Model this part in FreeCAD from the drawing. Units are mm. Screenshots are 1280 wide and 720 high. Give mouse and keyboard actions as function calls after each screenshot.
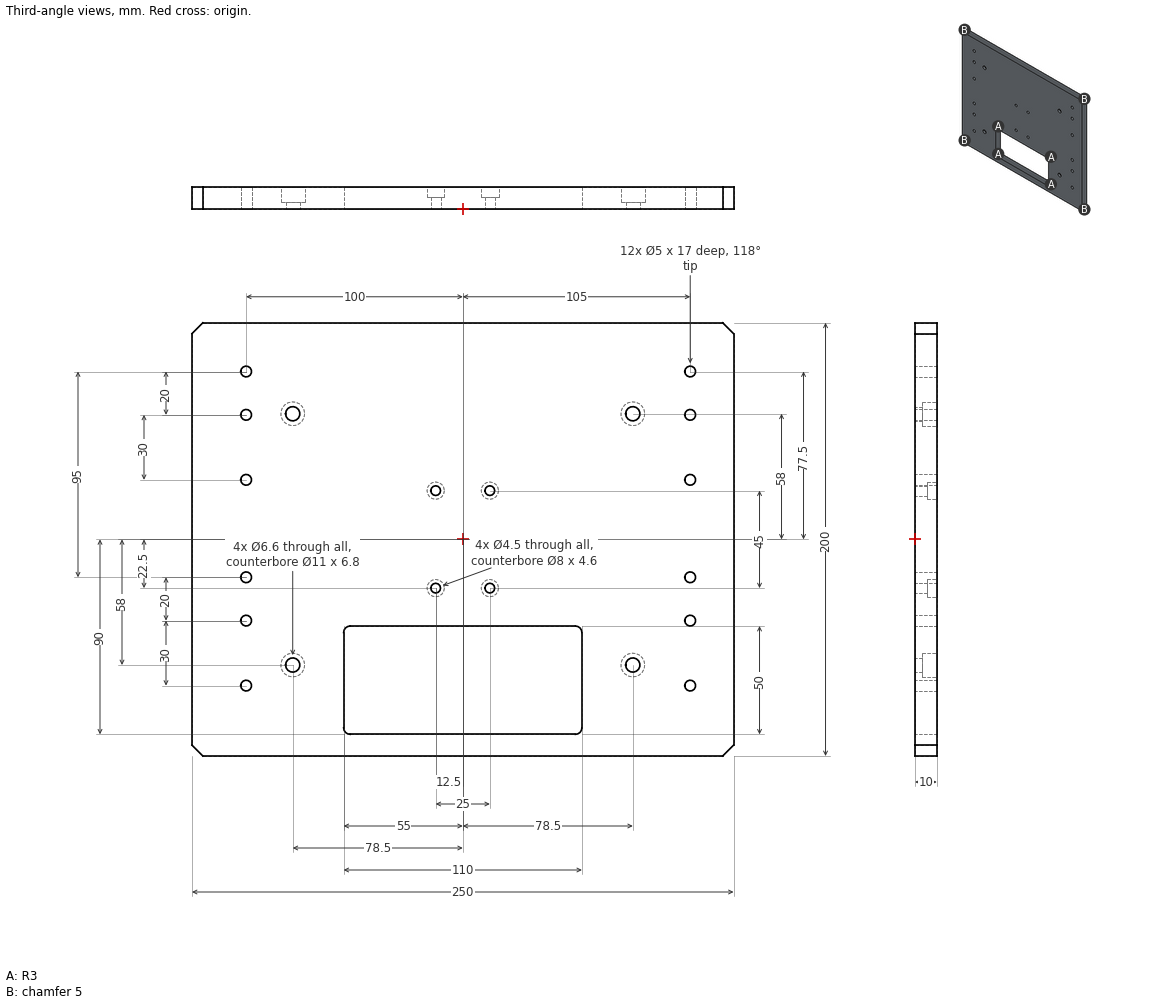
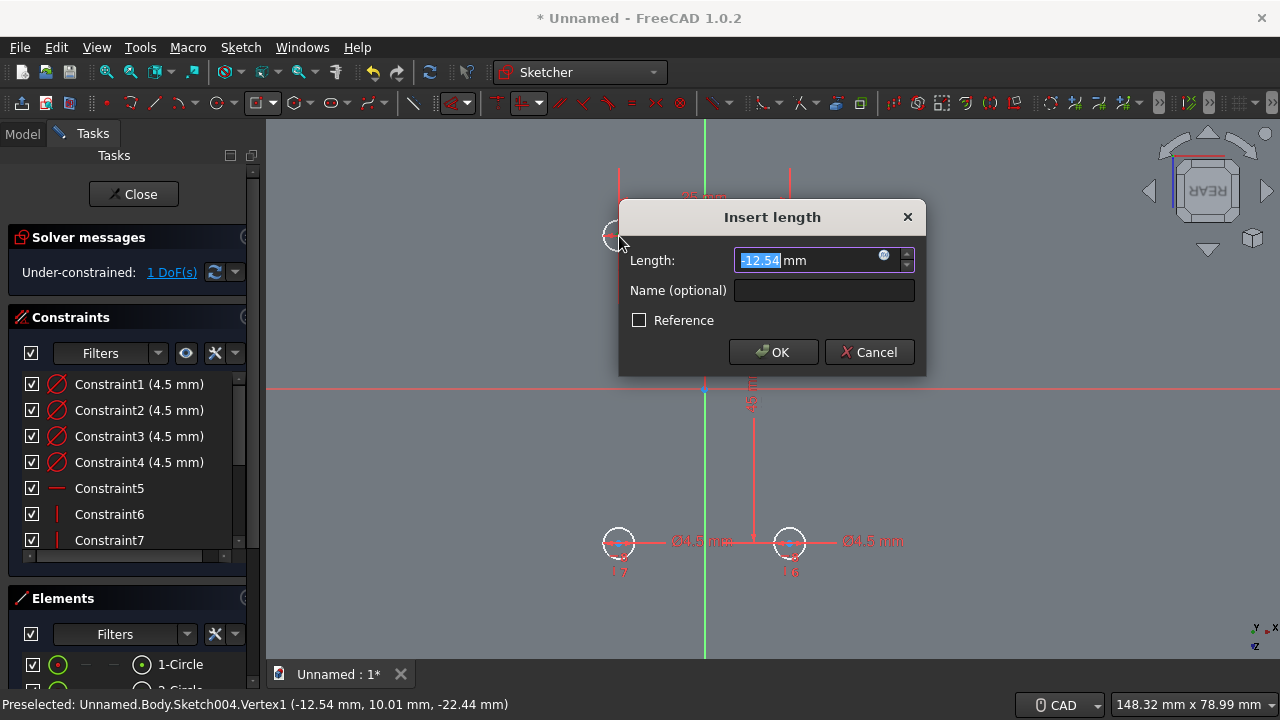
text(-12.5)
key(Return)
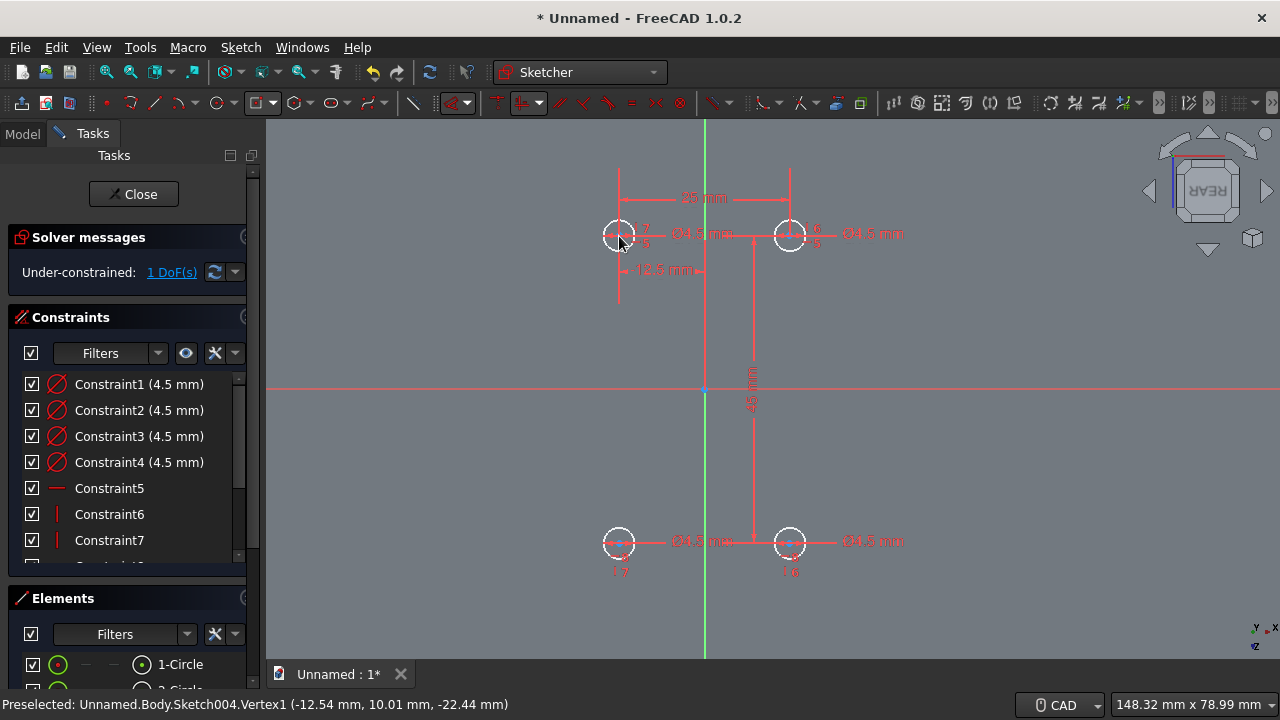
click(619, 236)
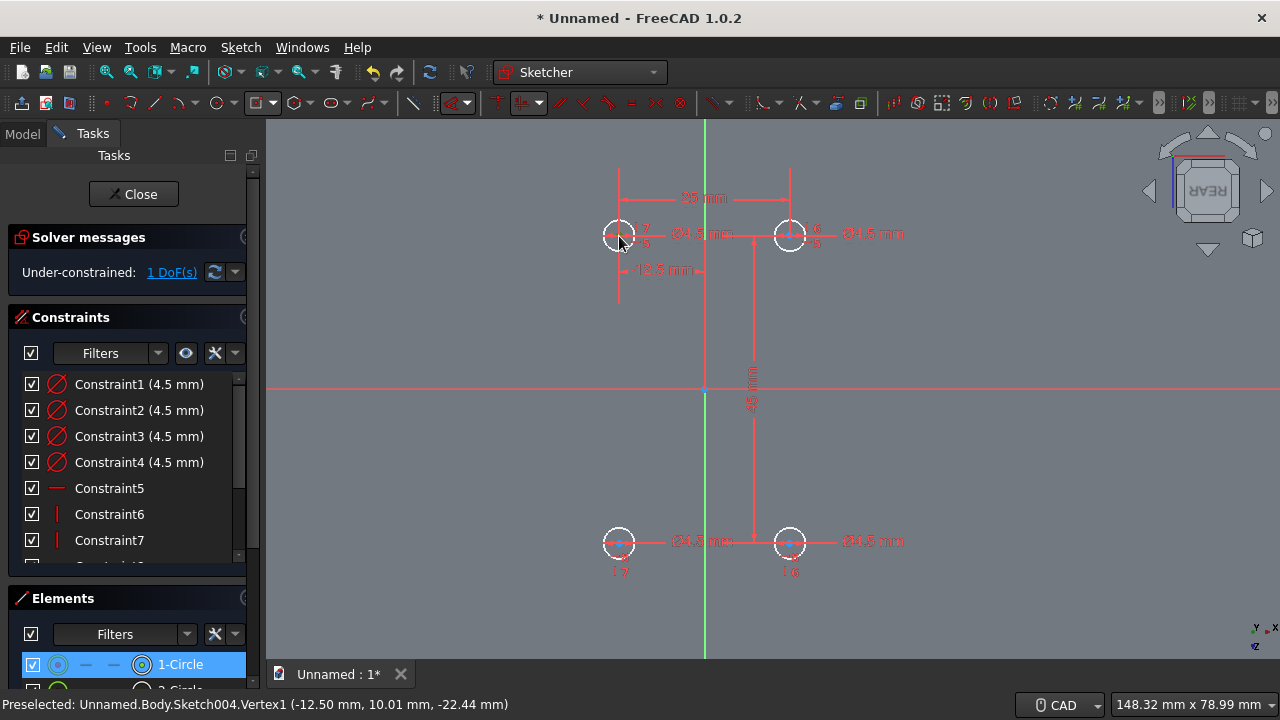
key(i)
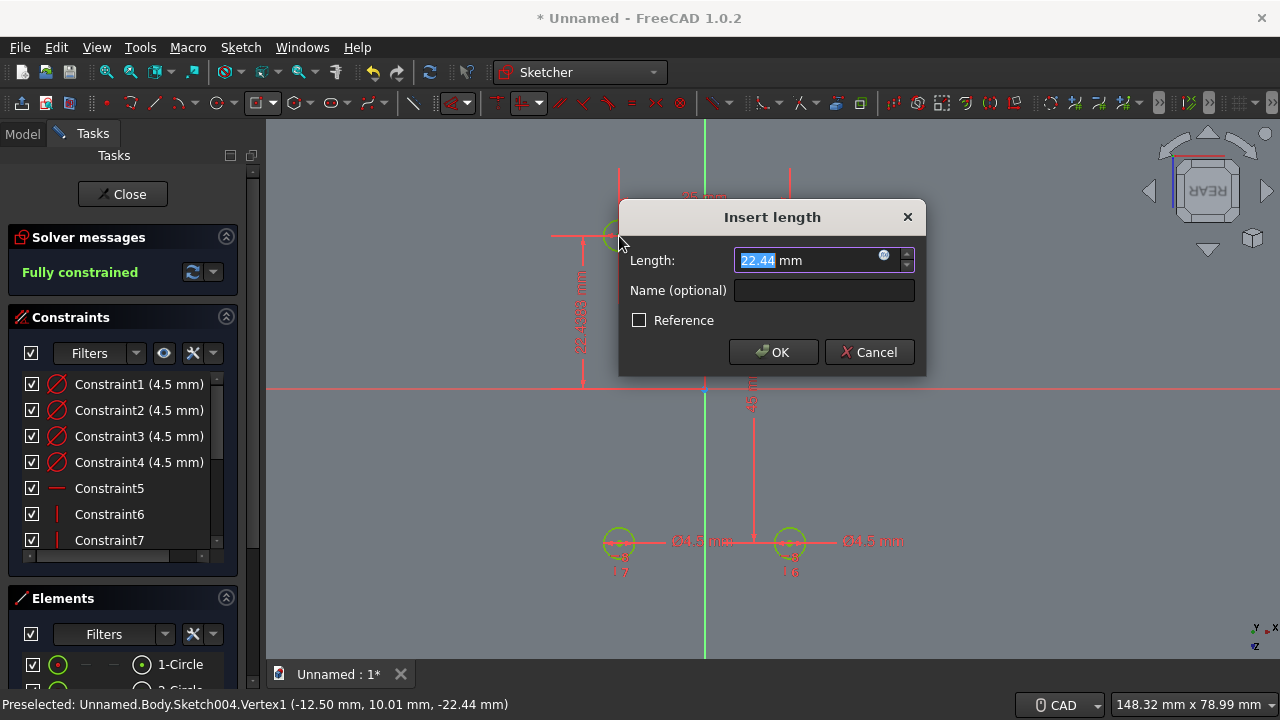
text(22.5)
key(Return)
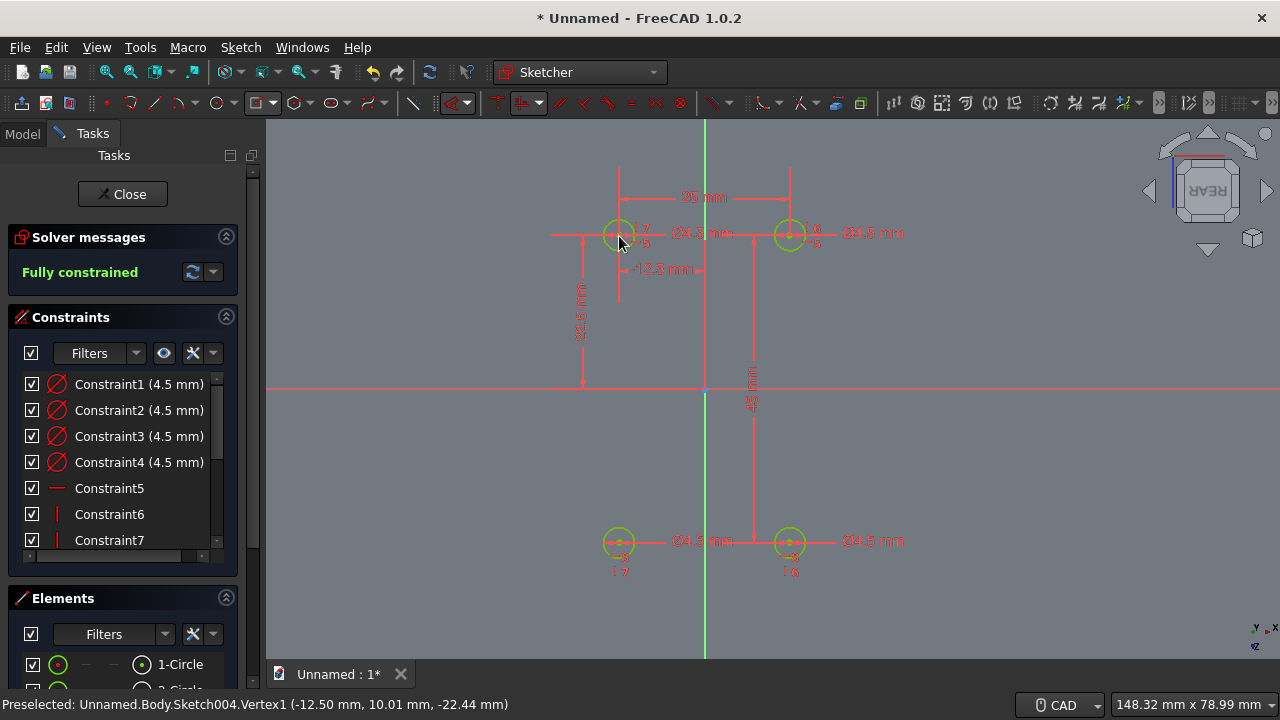
click(123, 194)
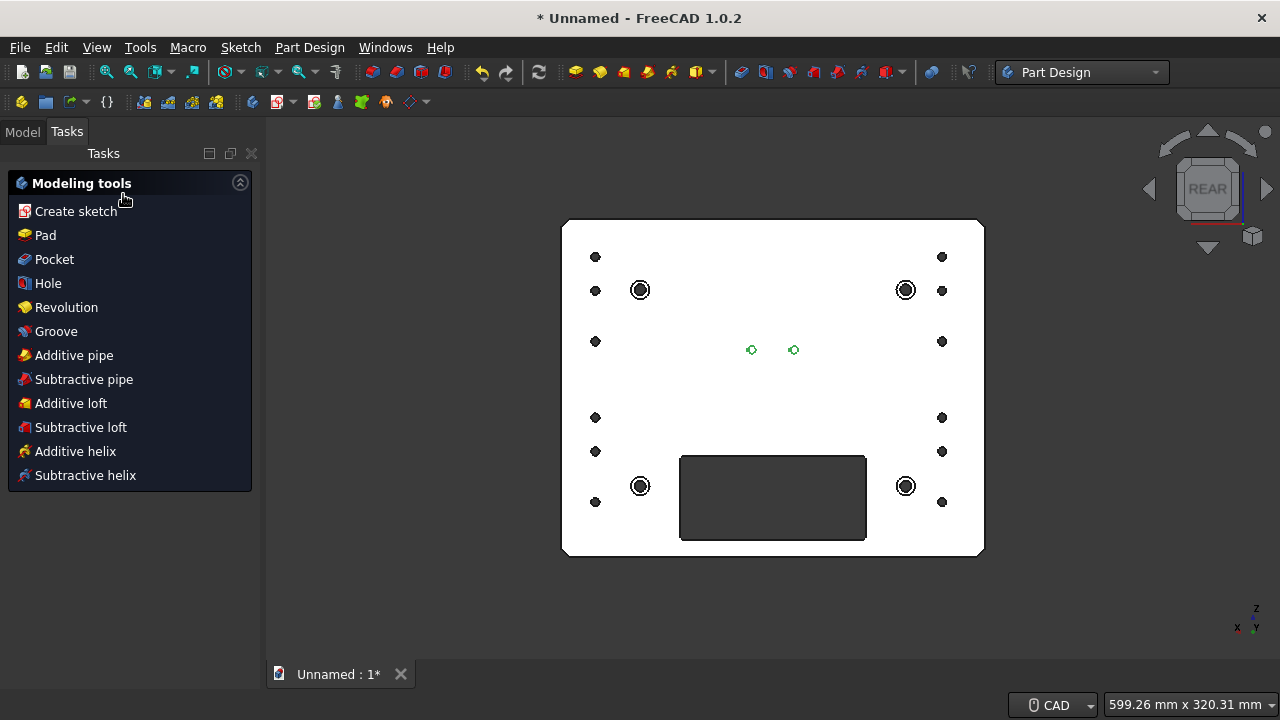
click(766, 72)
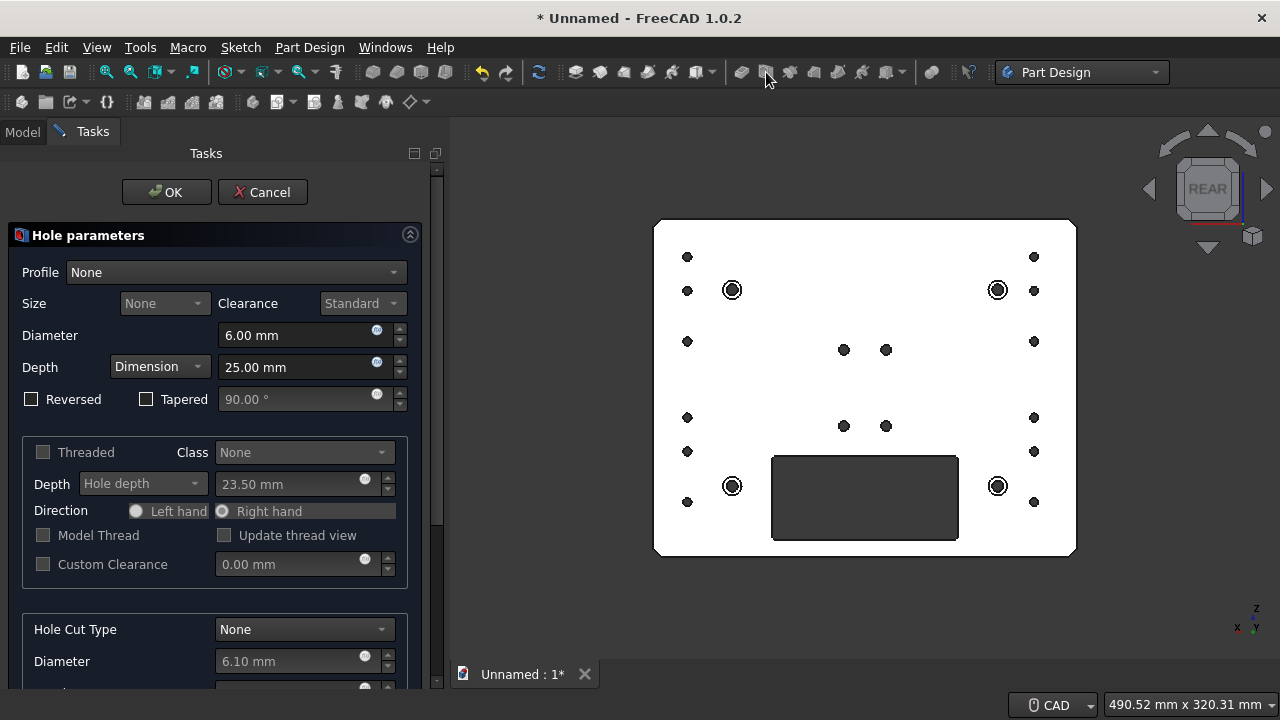
triple_click(305, 335)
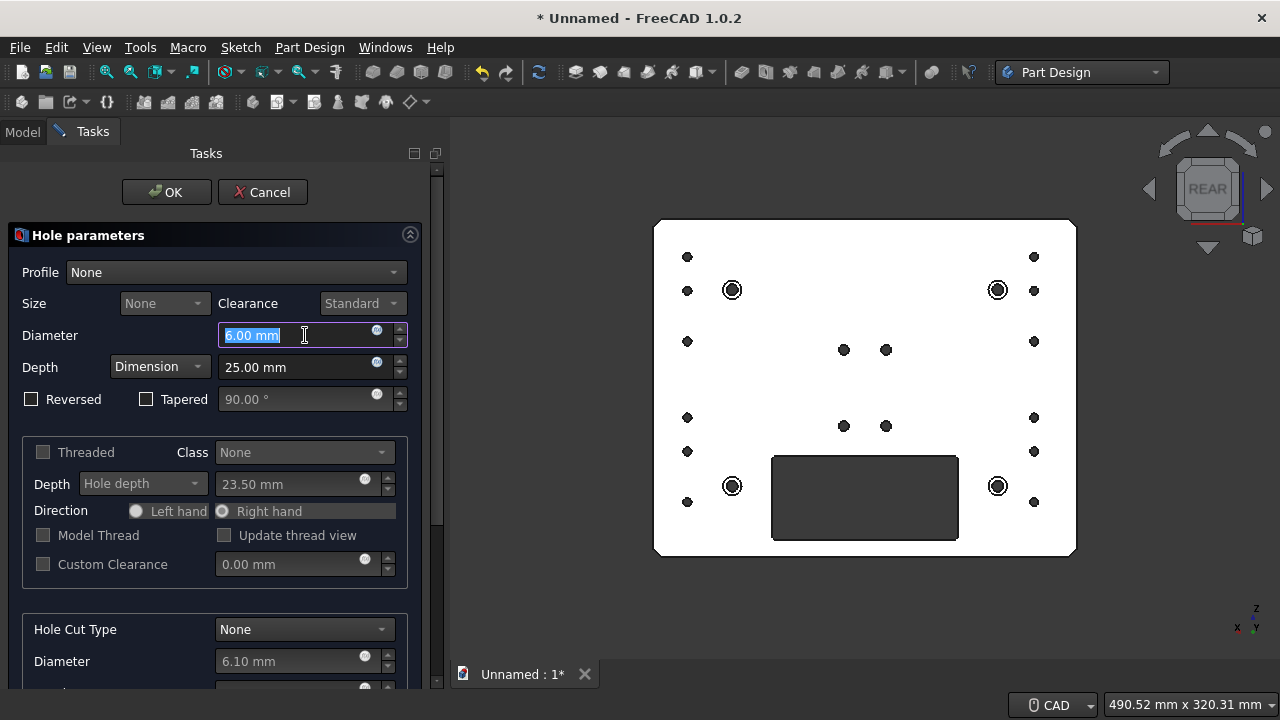
text(4.5)
key(Tab)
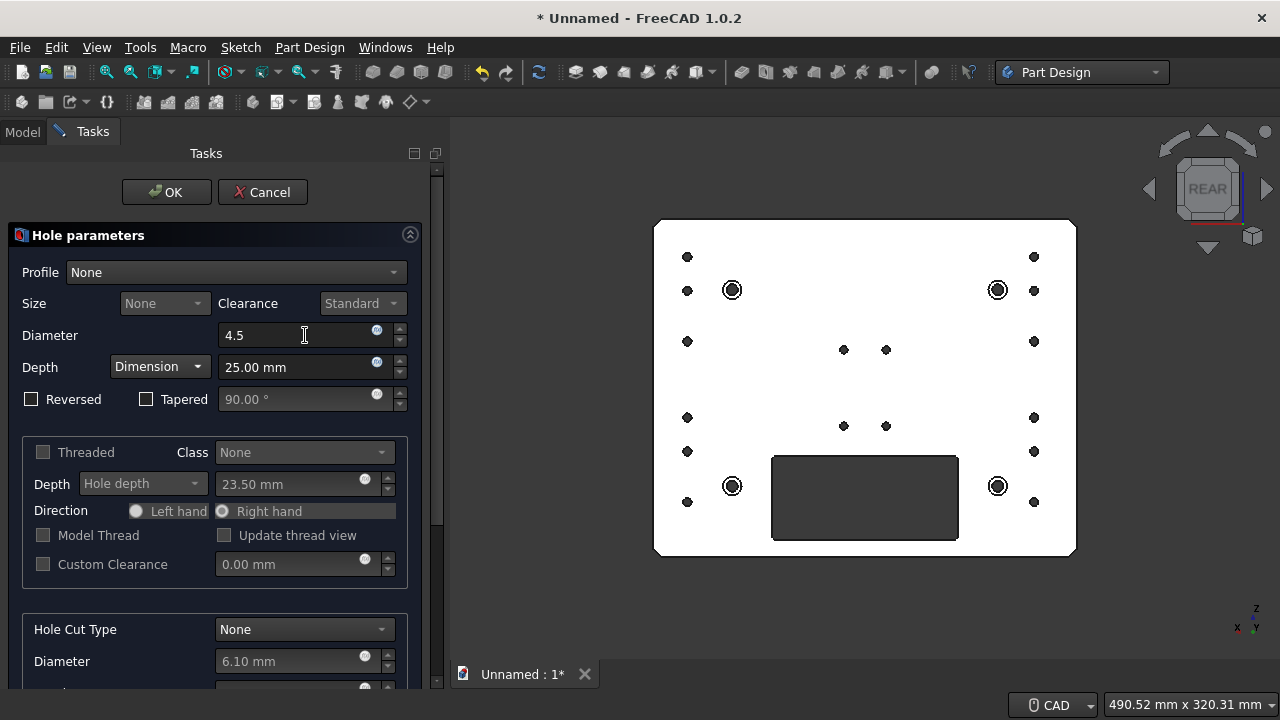
click(161, 366)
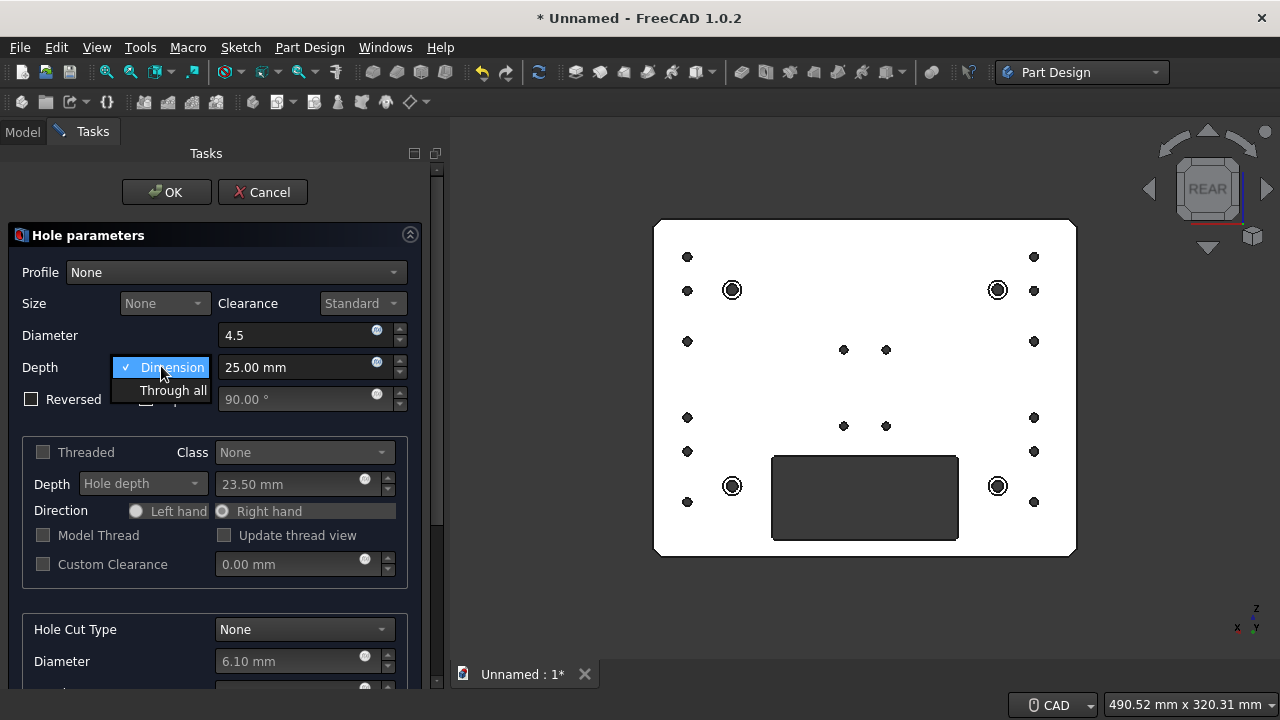
click(160, 390)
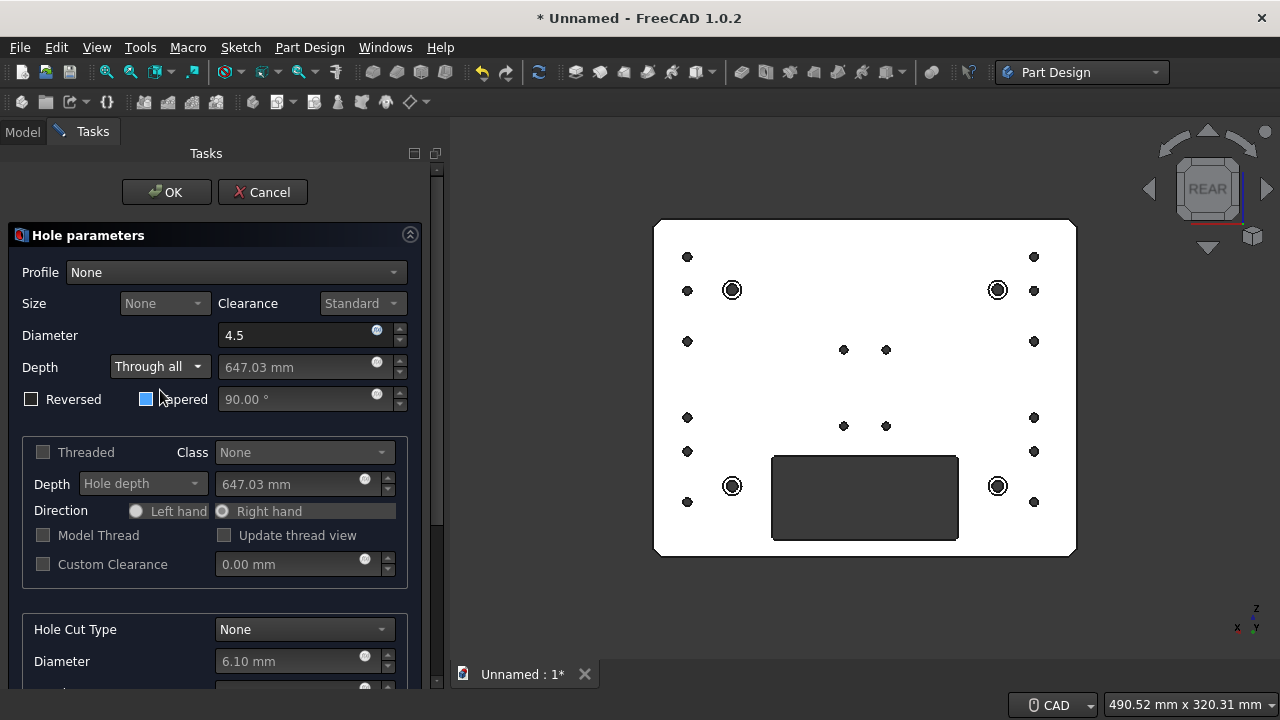
click(306, 630)